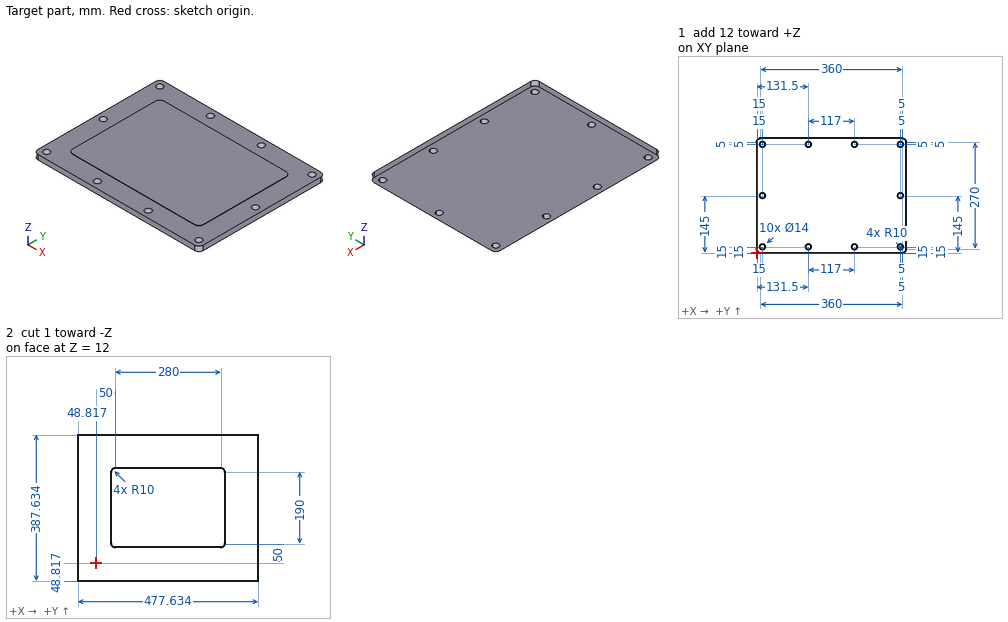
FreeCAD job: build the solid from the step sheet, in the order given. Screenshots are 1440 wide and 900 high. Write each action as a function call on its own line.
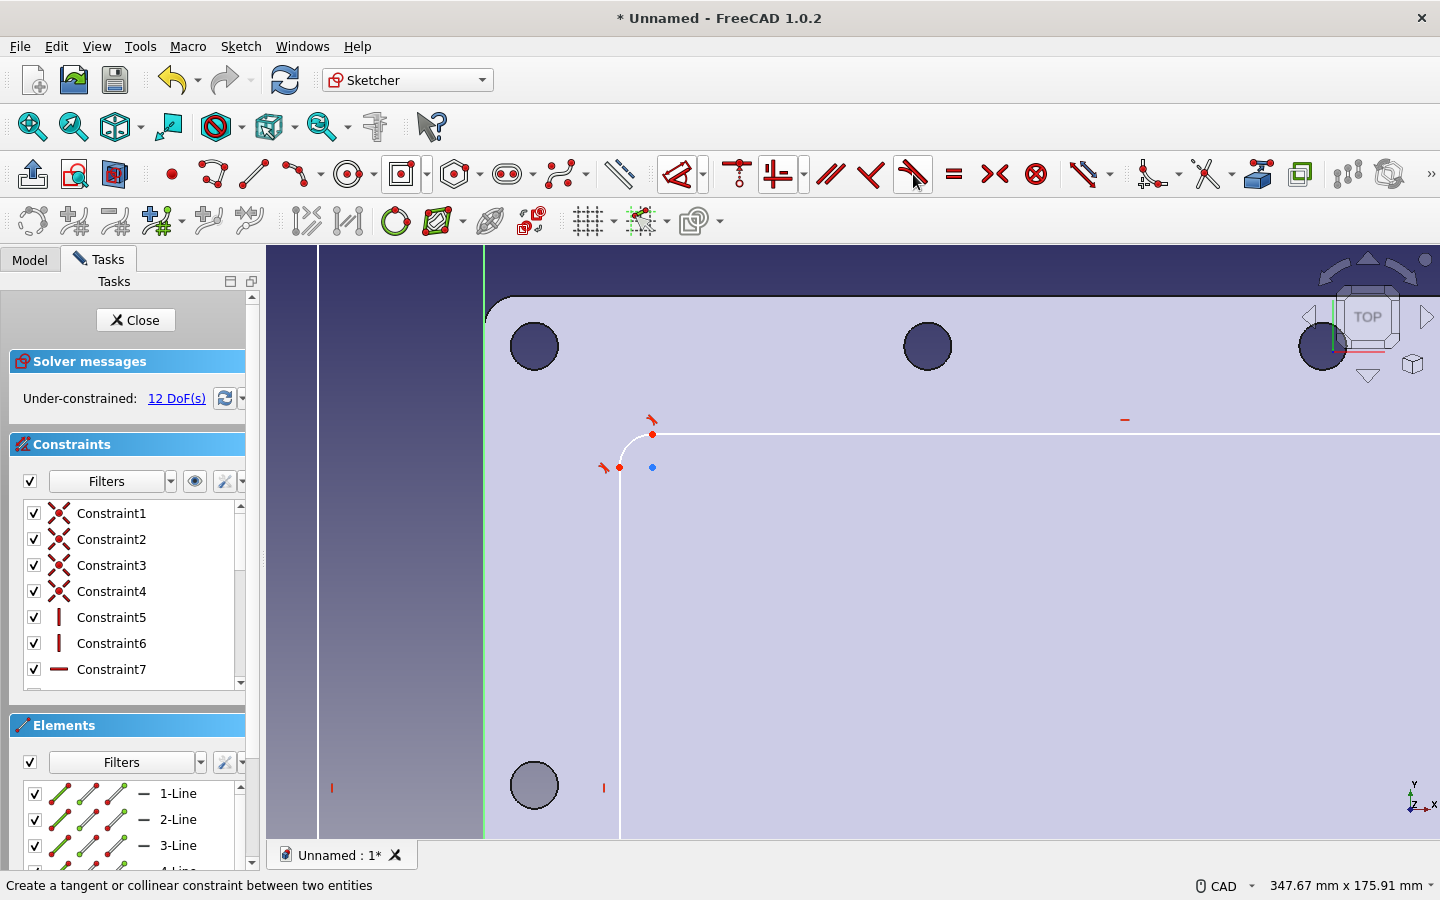
scroll(638, 437, down, 6)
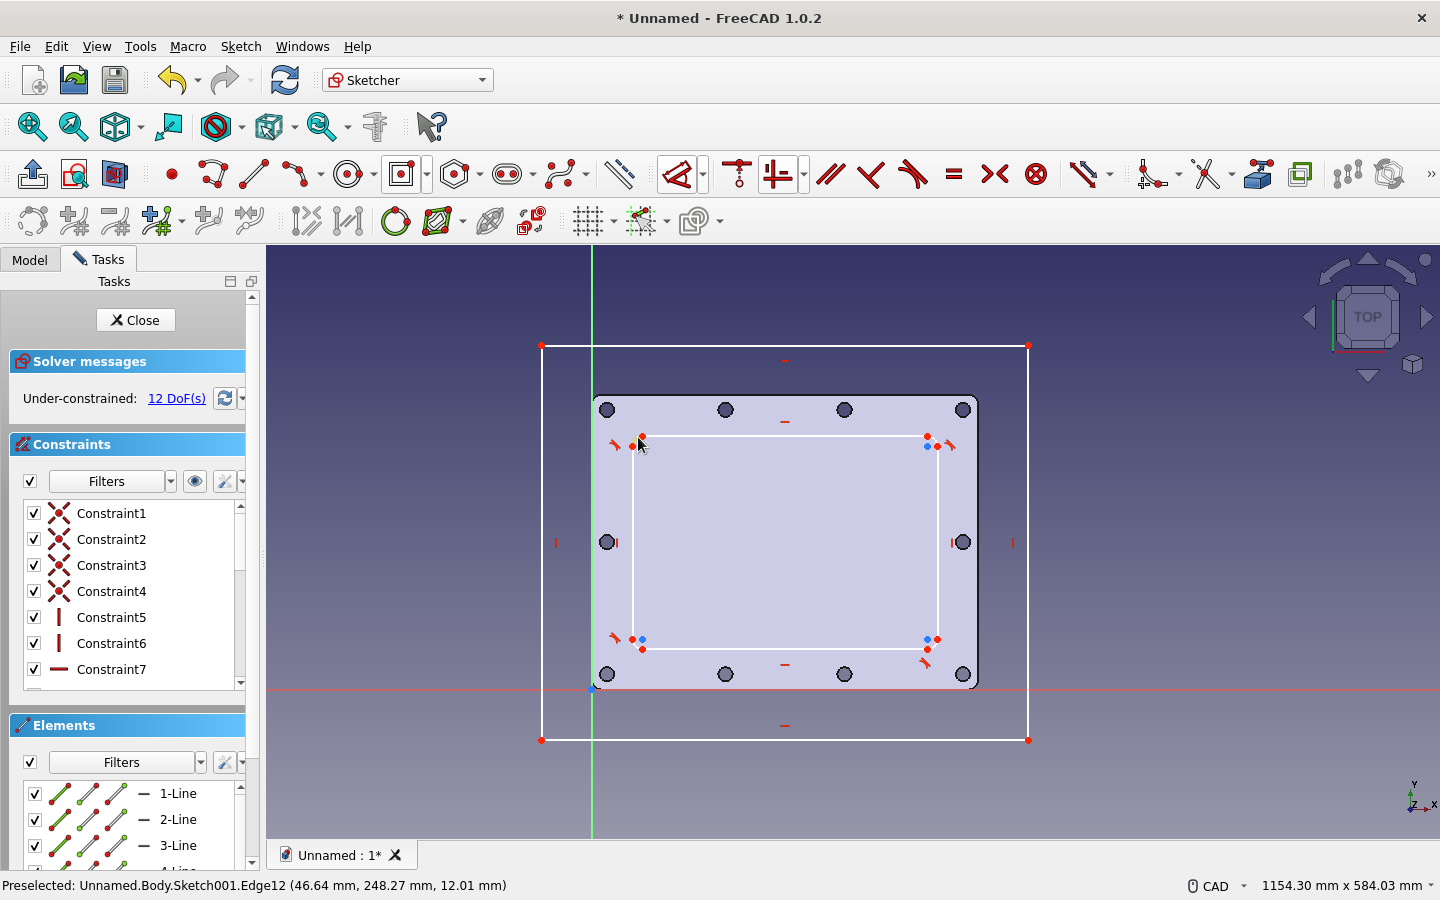
scroll(937, 442, up, 6)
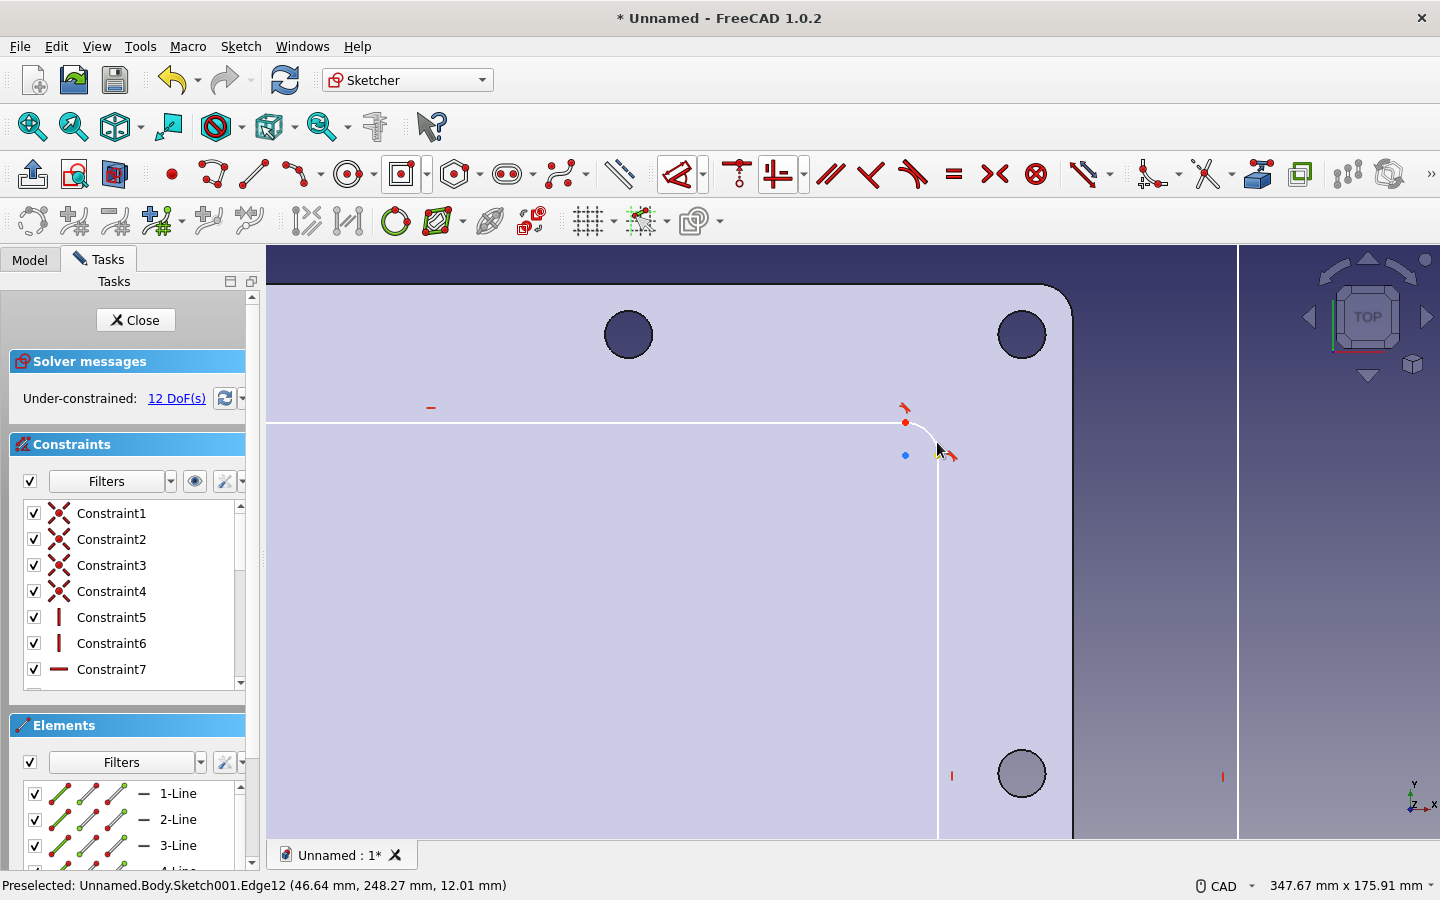
click(934, 441)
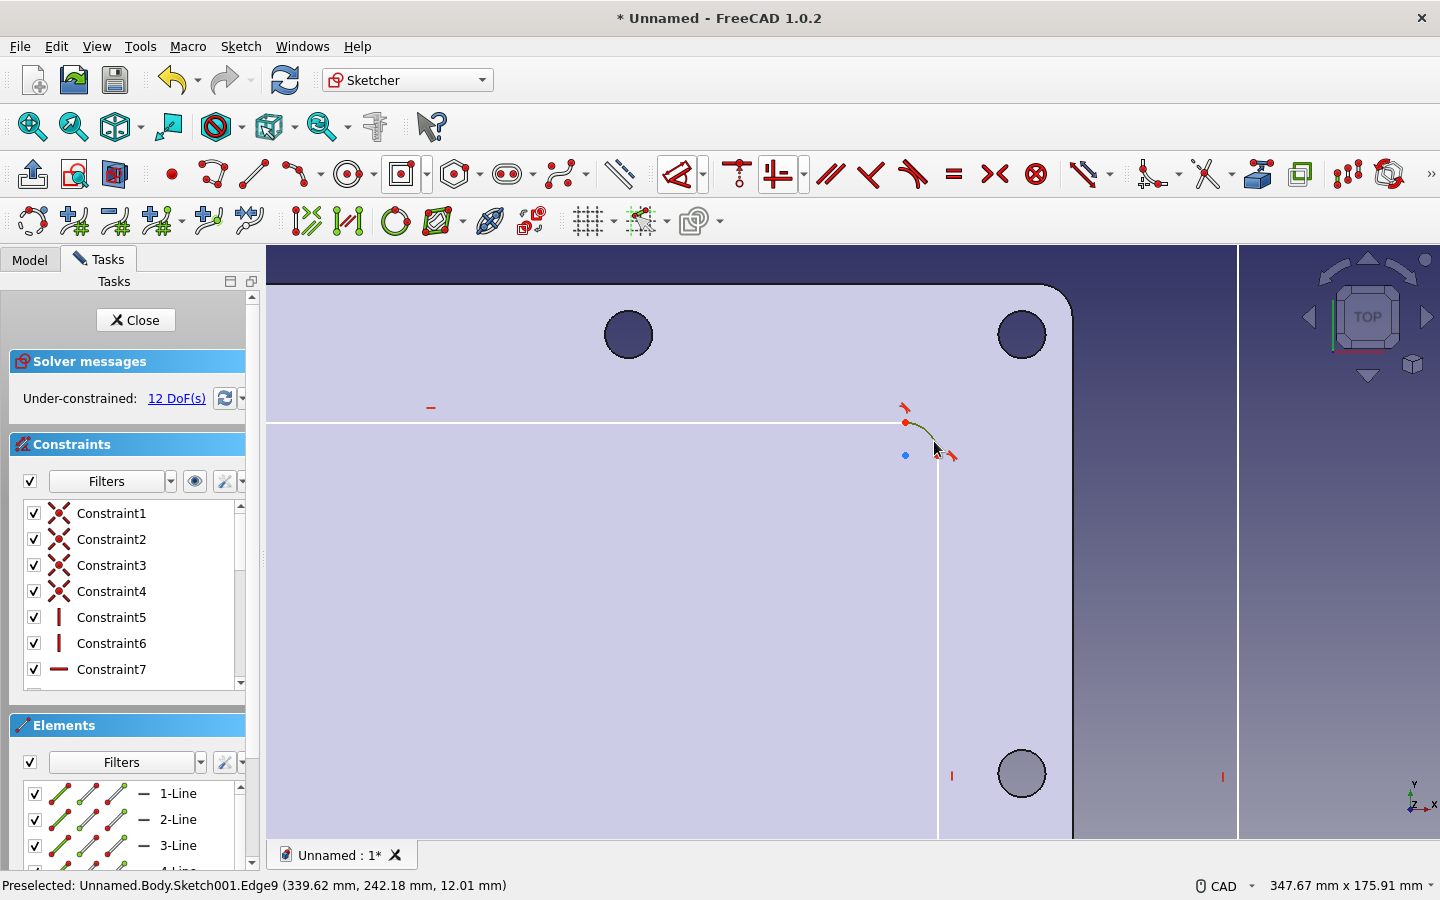
scroll(937, 442, down, 6)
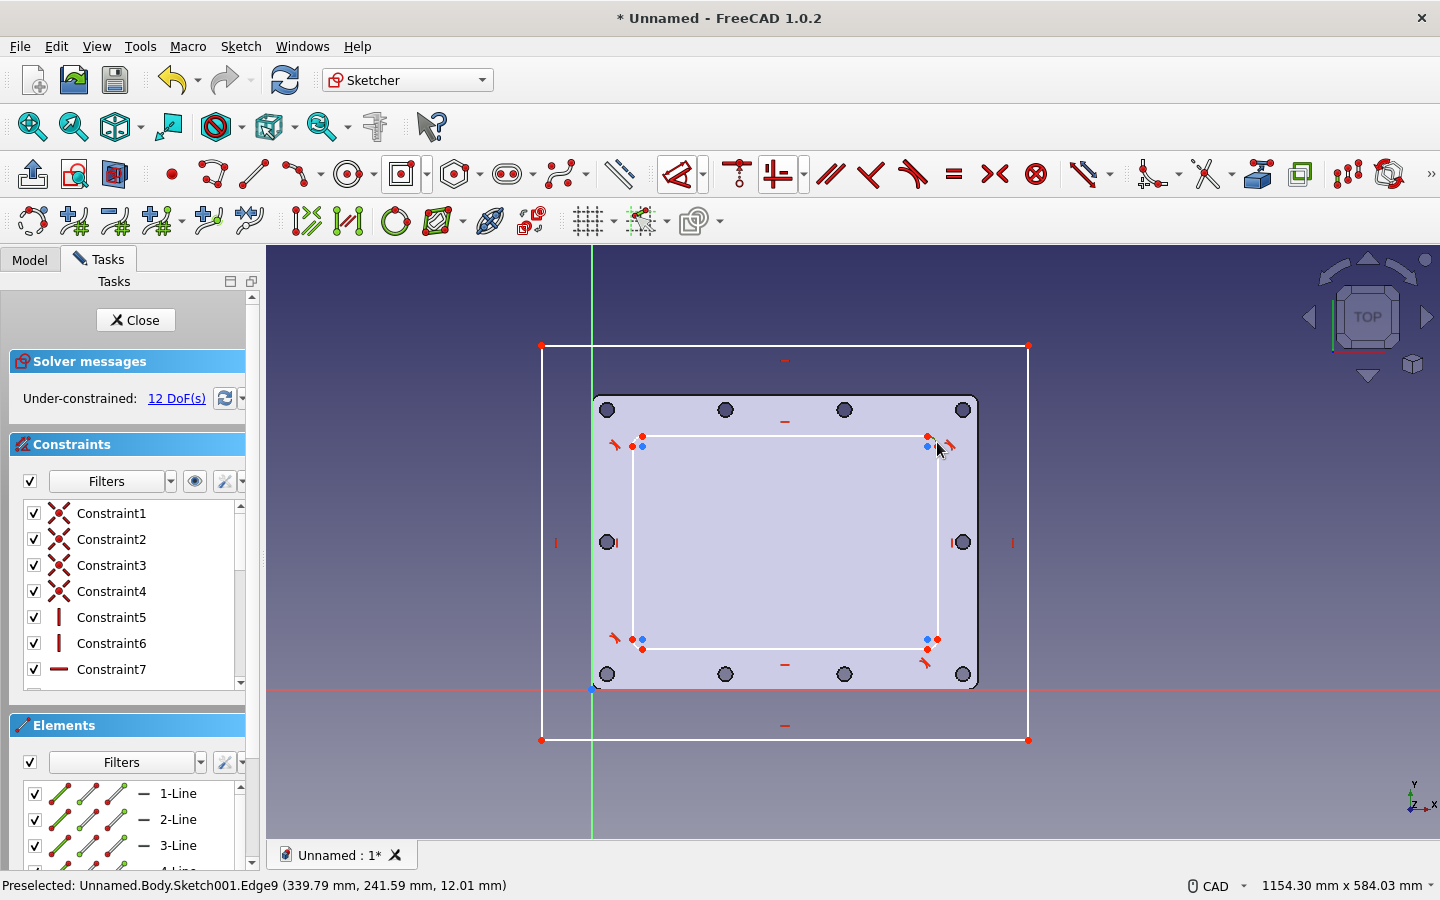
scroll(932, 648, up, 6)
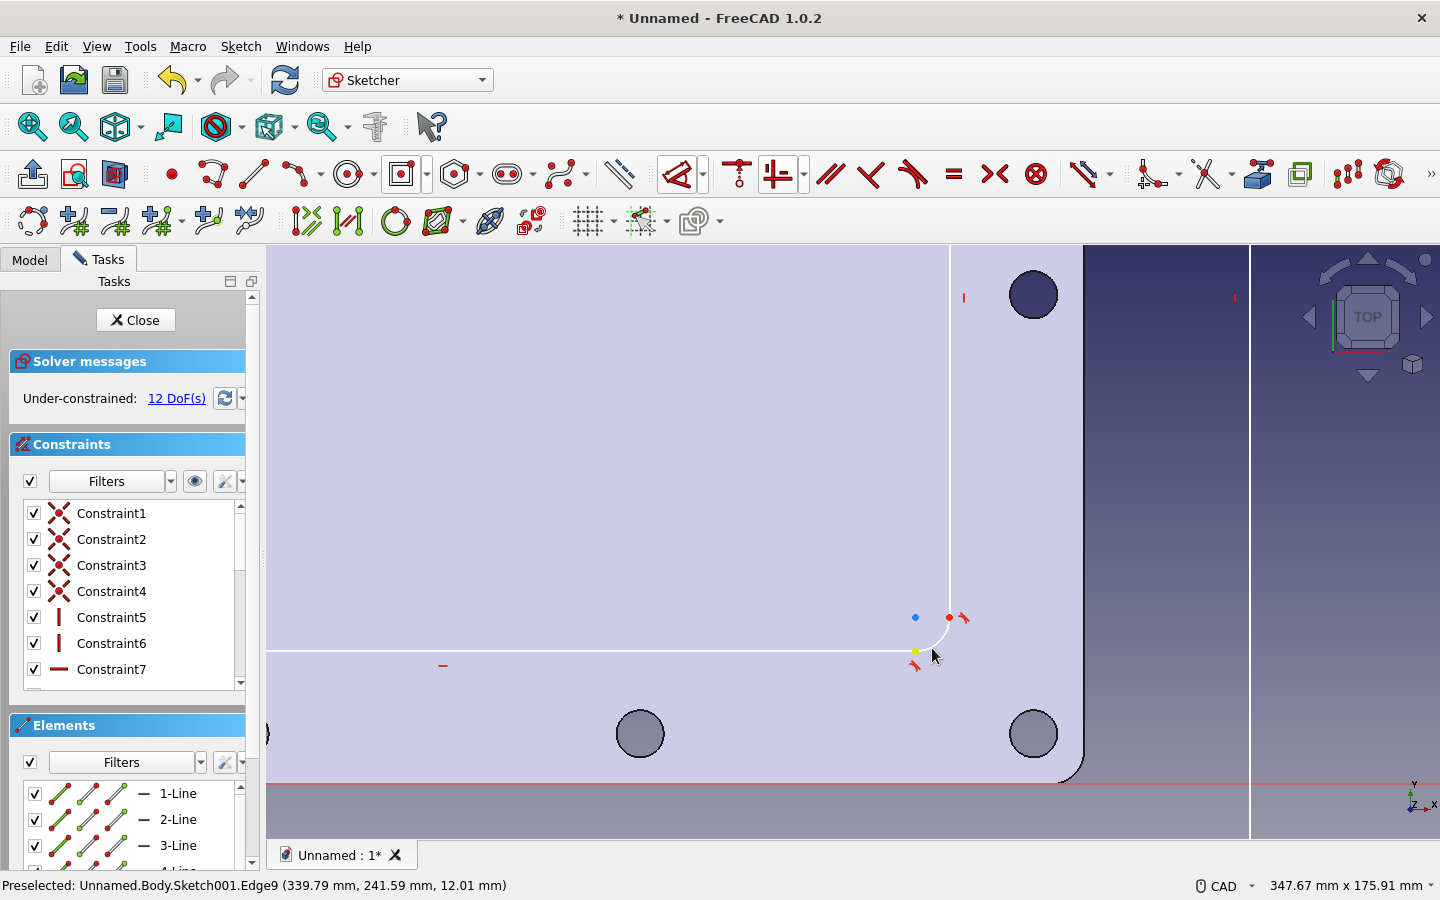
click(931, 647)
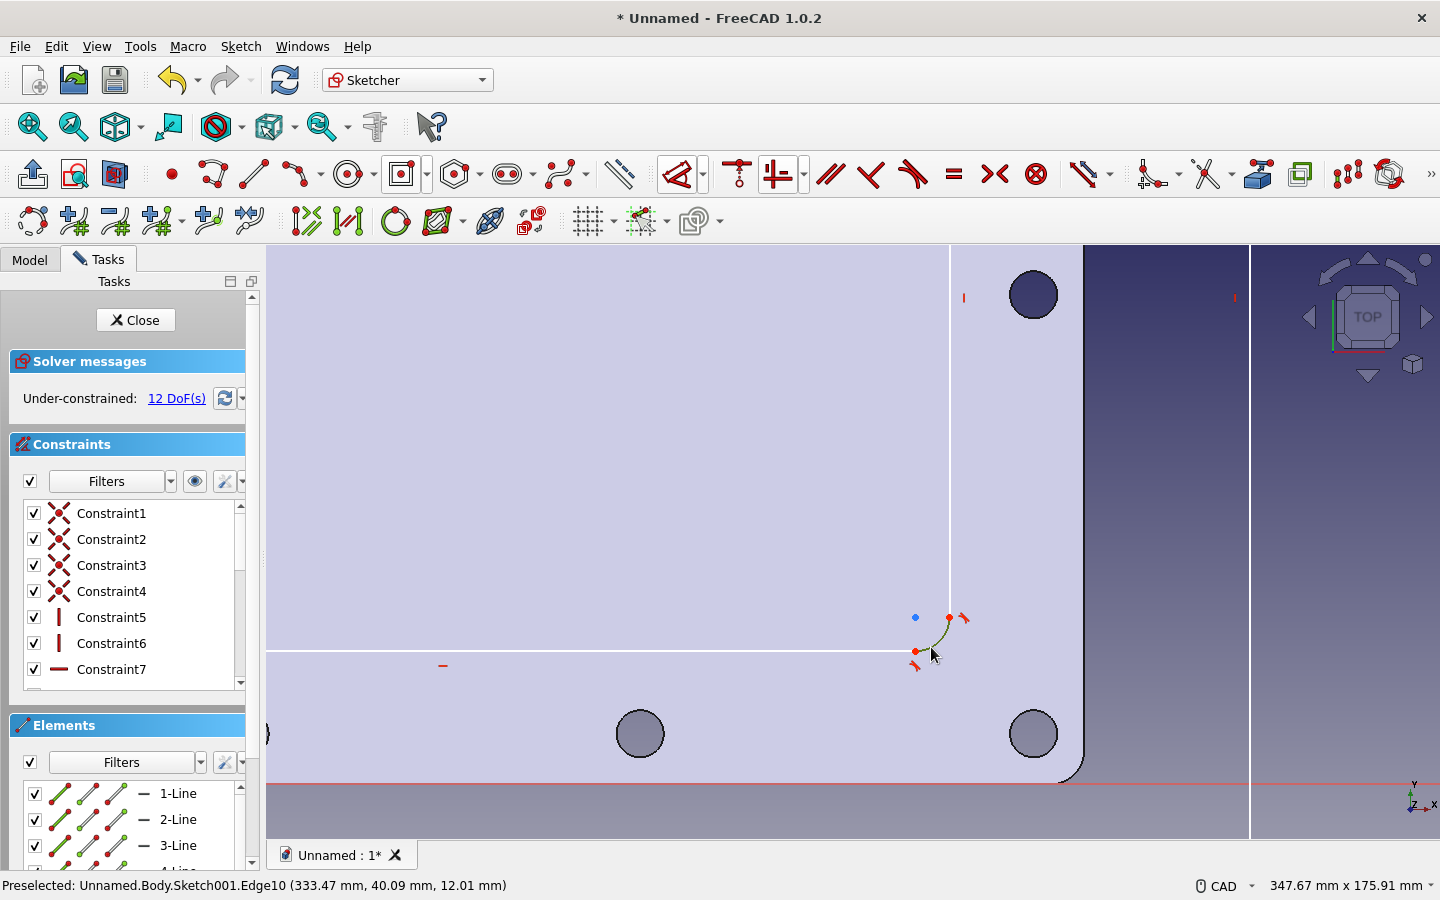
scroll(932, 649, down, 6)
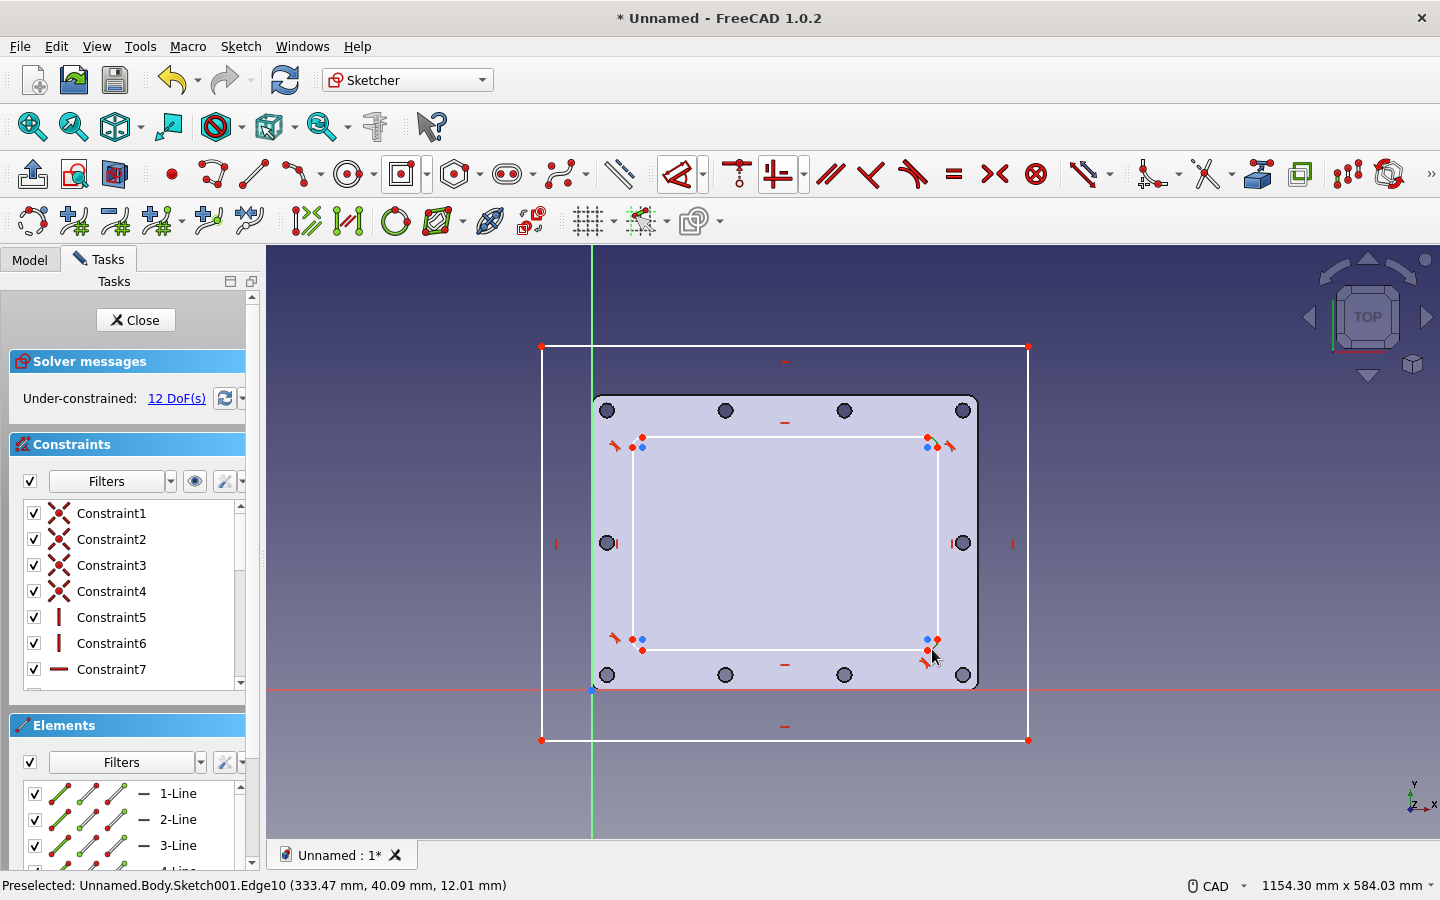
scroll(634, 645, up, 6)